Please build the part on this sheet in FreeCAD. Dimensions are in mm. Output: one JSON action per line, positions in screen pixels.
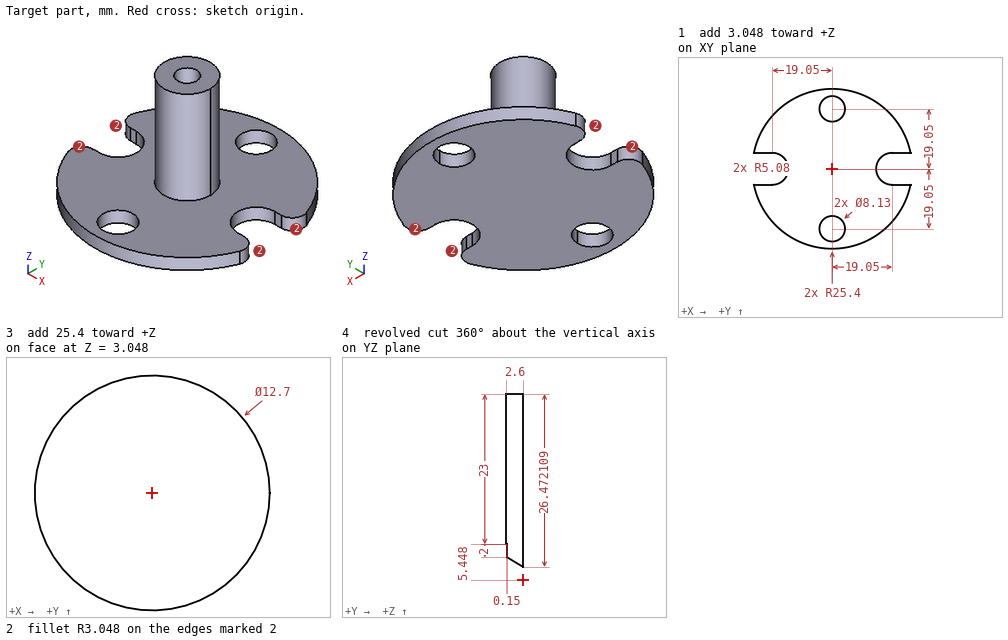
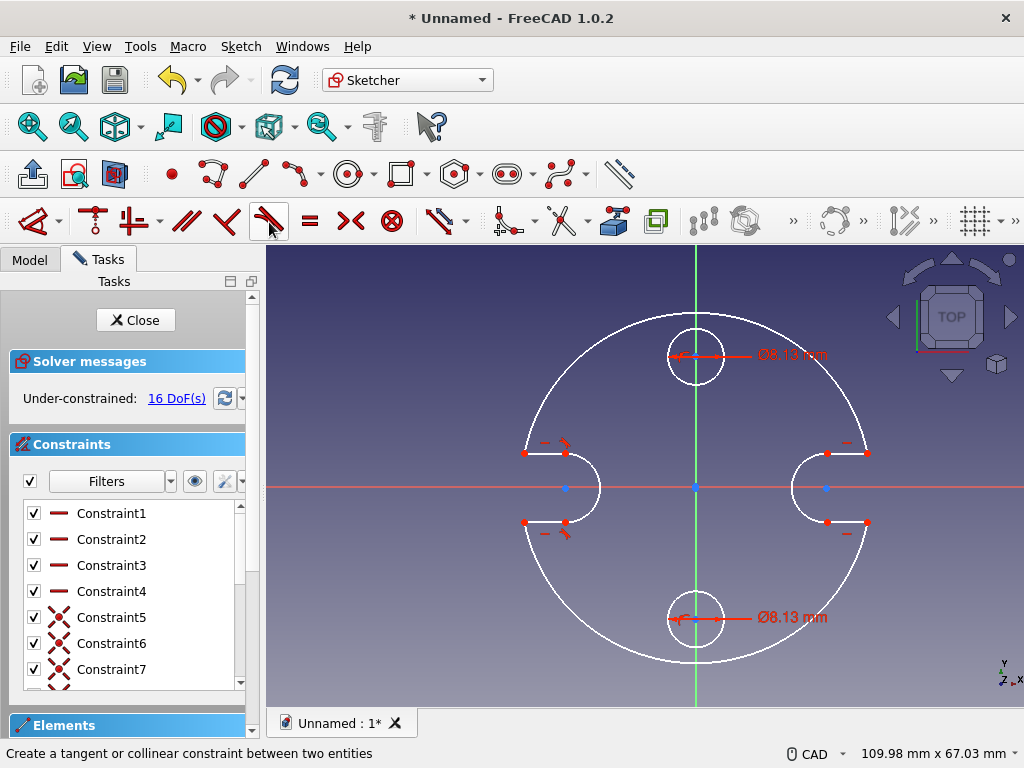
{"action": "left_click", "coordinate": [855, 522]}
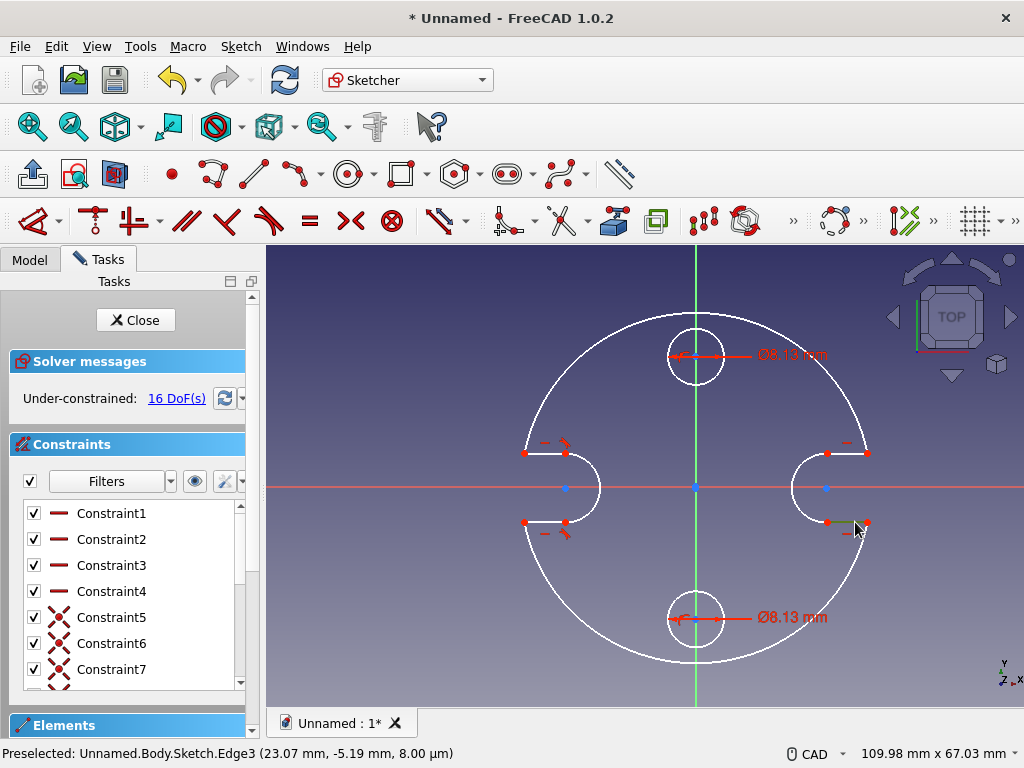
{"action": "left_click", "coordinate": [799, 468]}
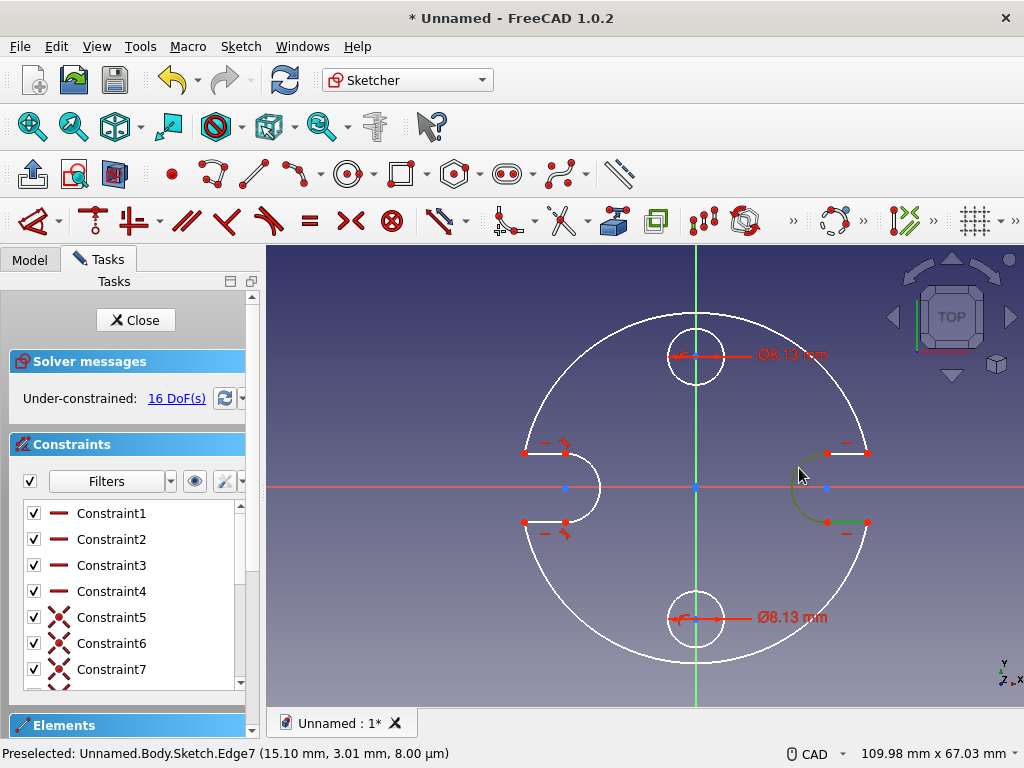
{"action": "left_click", "coordinate": [269, 222]}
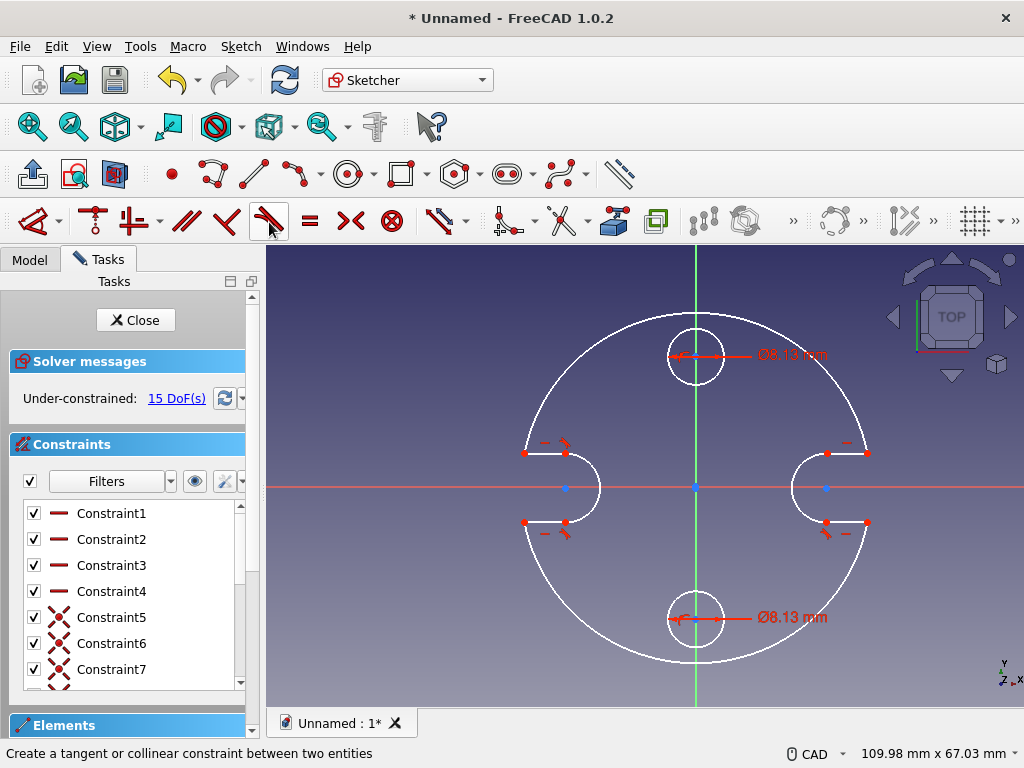
{"action": "left_click", "coordinate": [839, 454]}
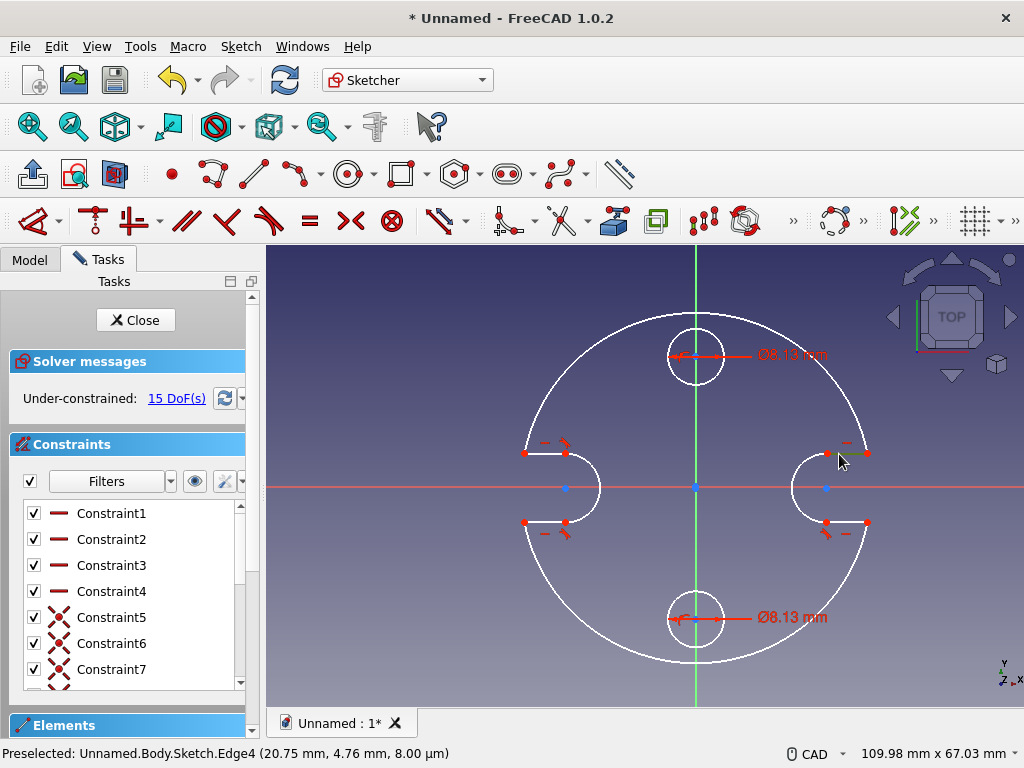
{"action": "left_click", "coordinate": [799, 467]}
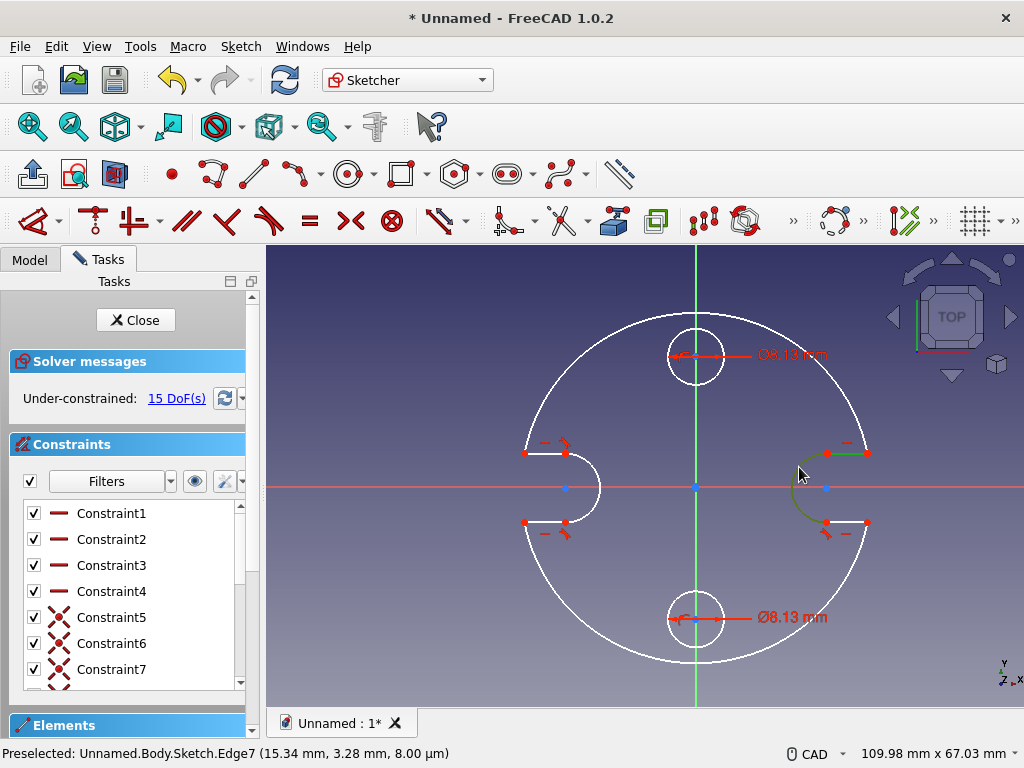
{"action": "left_click", "coordinate": [269, 222]}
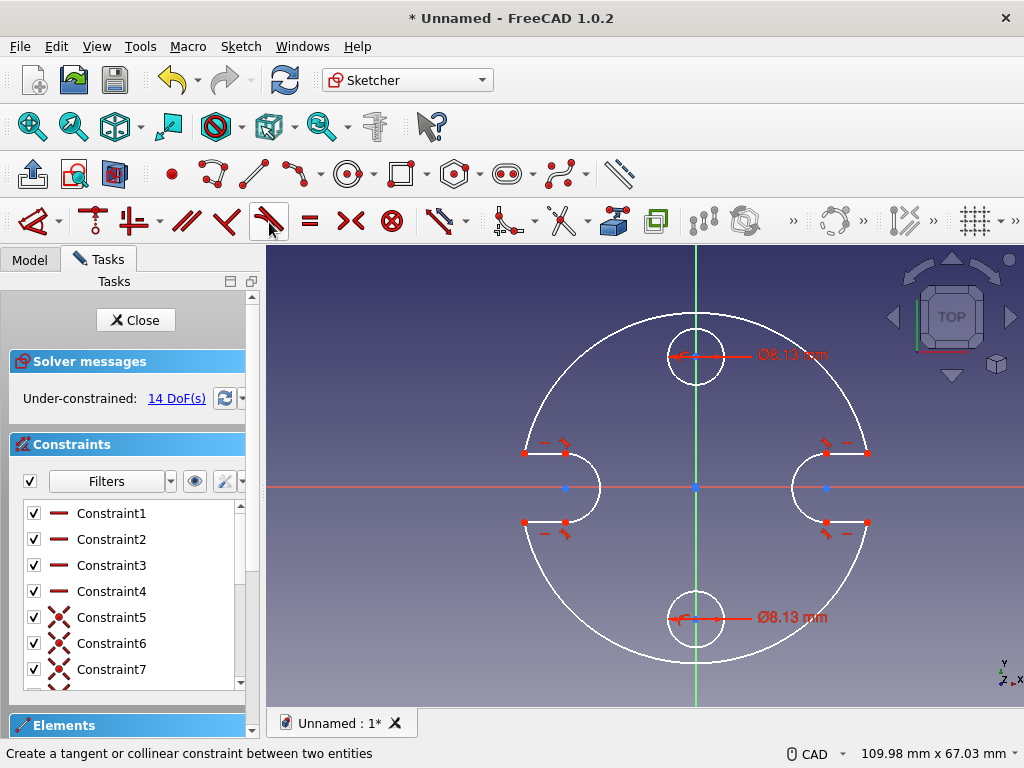
{"action": "left_click", "coordinate": [605, 638]}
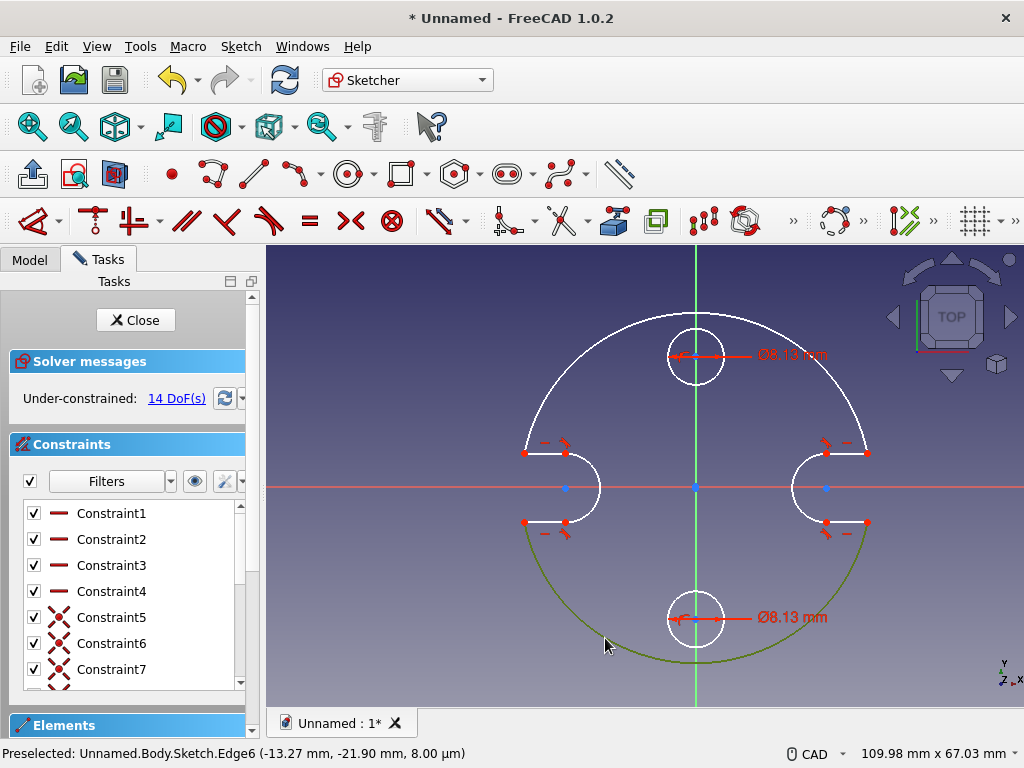
{"action": "left_click", "coordinate": [787, 339]}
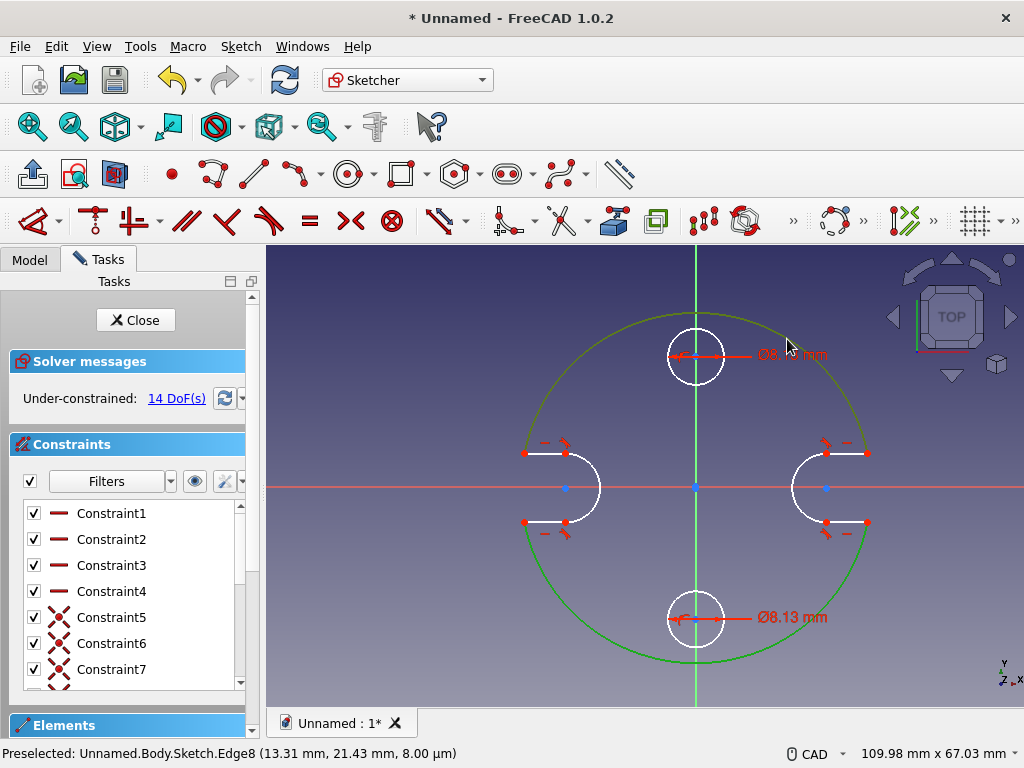
{"action": "left_click", "coordinate": [93, 222]}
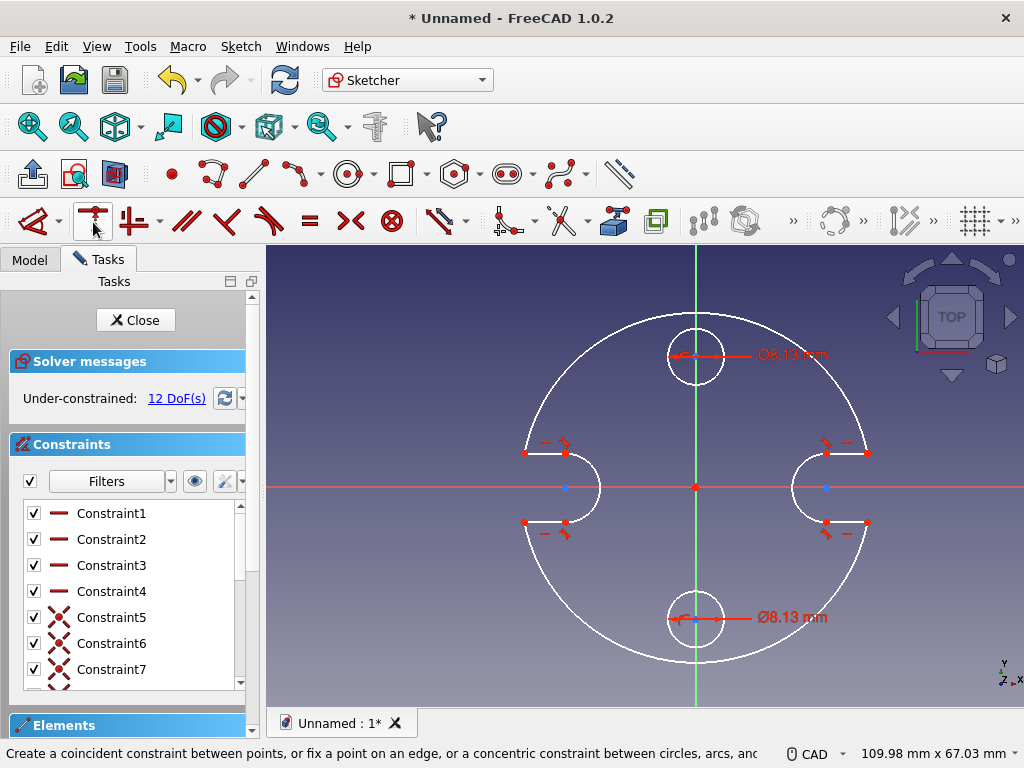
{"action": "scroll", "coordinate": [696, 487], "scroll_direction": "up", "scroll_amount": 2}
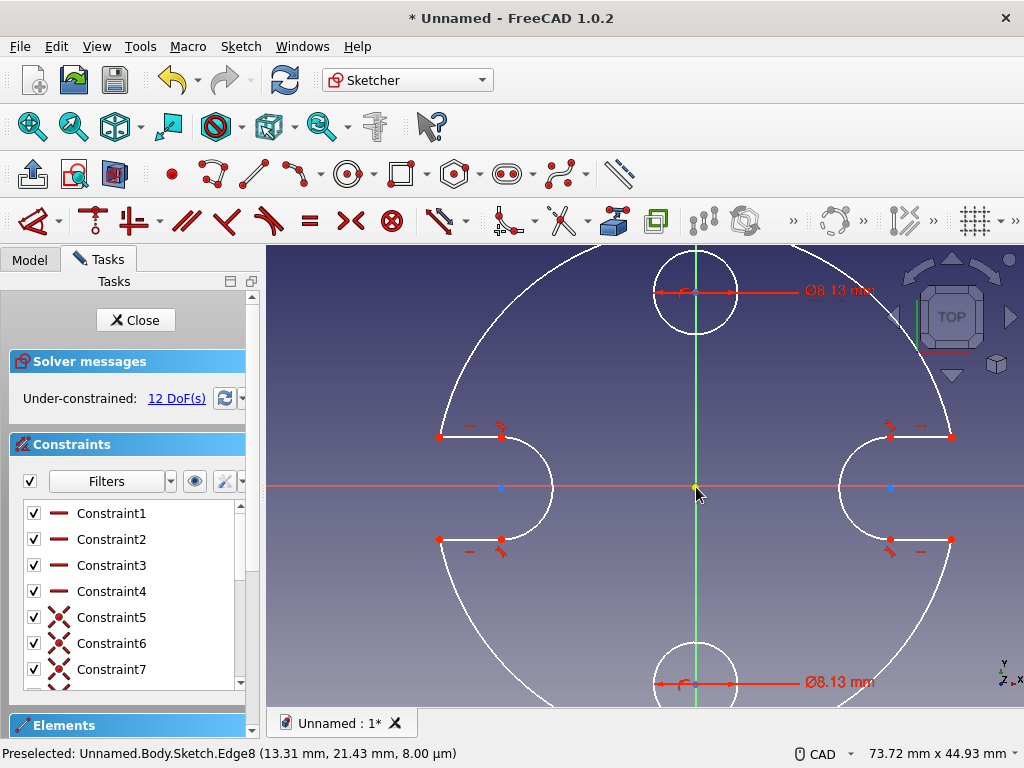
{"action": "left_click_drag", "start_coordinate": [686, 476], "coordinate": [706, 498]}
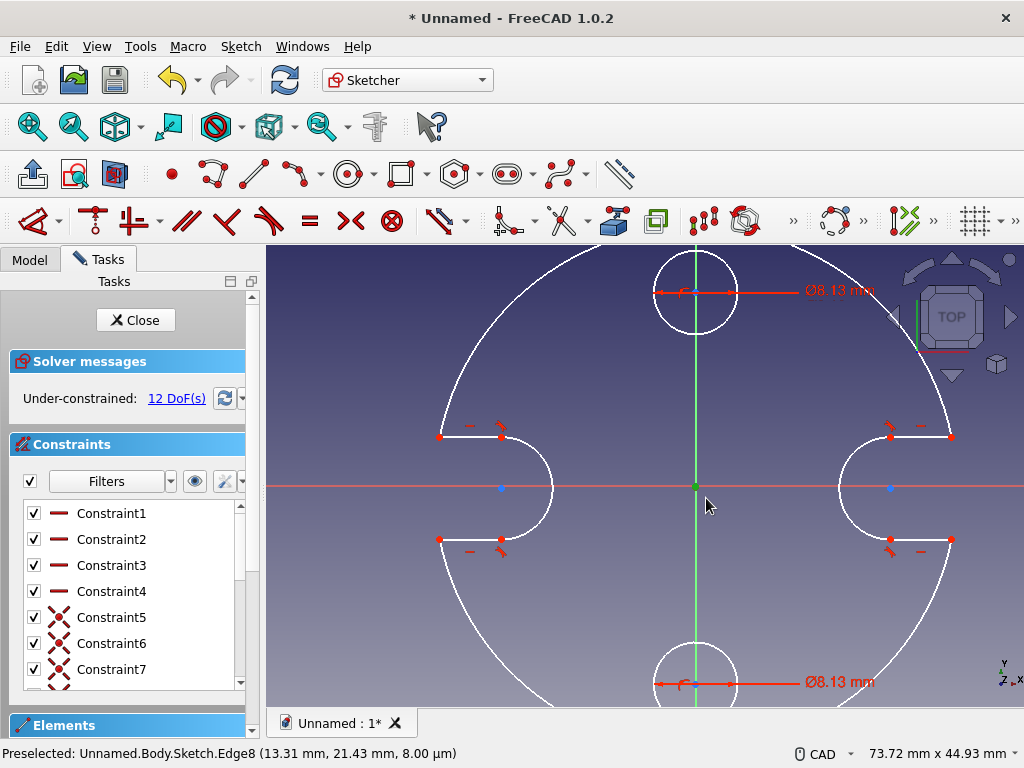
{"action": "left_click", "coordinate": [93, 222]}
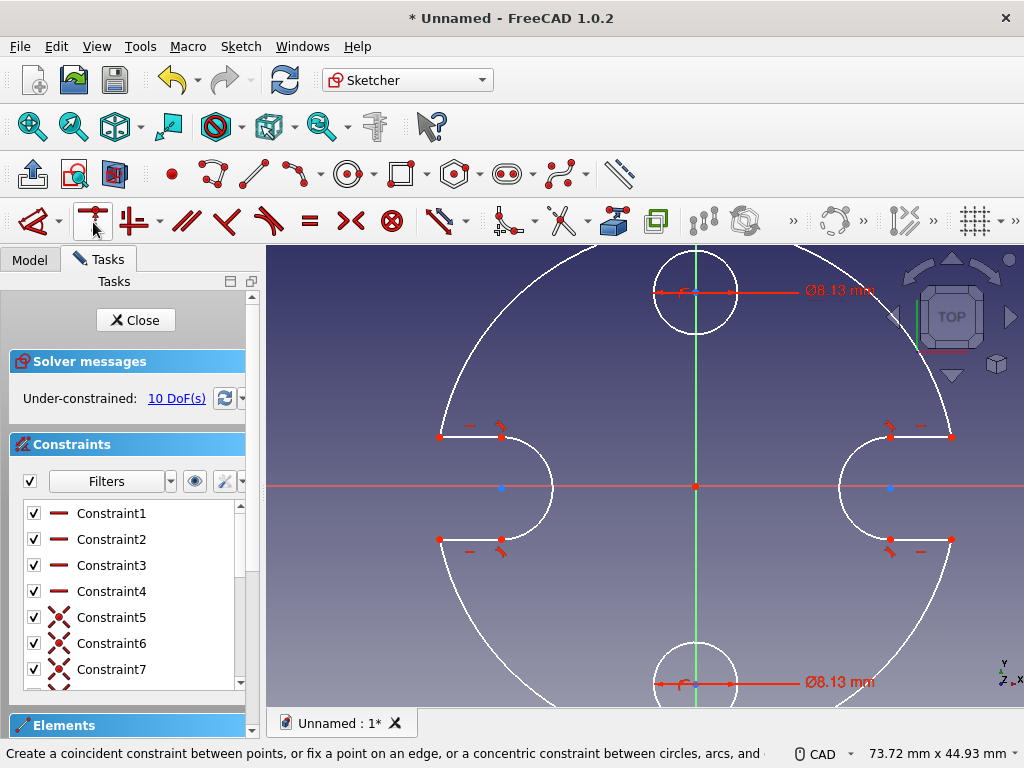
{"action": "left_click", "coordinate": [543, 518]}